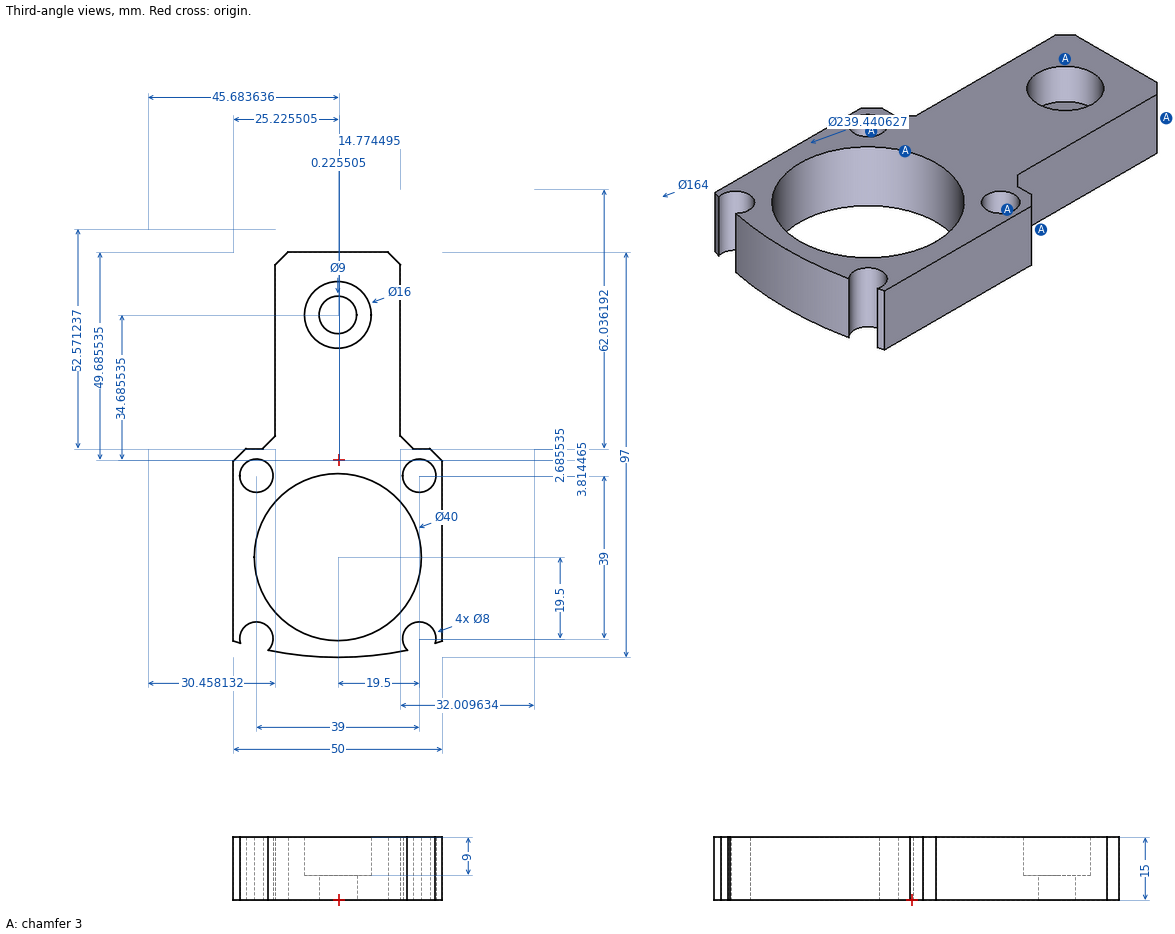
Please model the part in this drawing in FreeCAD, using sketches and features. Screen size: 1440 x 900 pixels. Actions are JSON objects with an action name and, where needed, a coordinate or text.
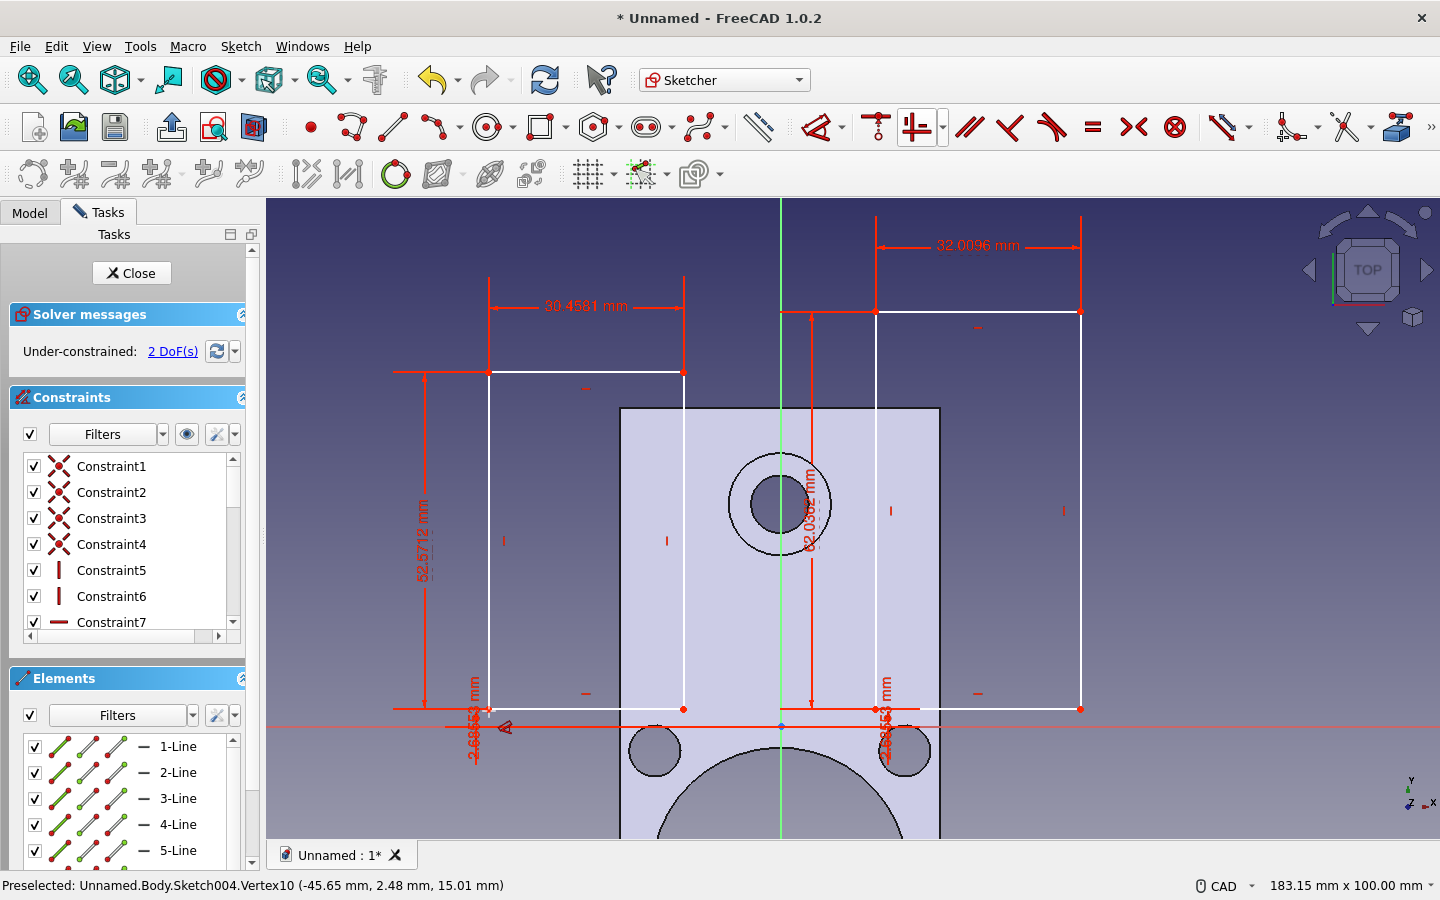
{"action": "left_click", "coordinate": [876, 312]}
{"action": "left_click", "coordinate": [828, 278]}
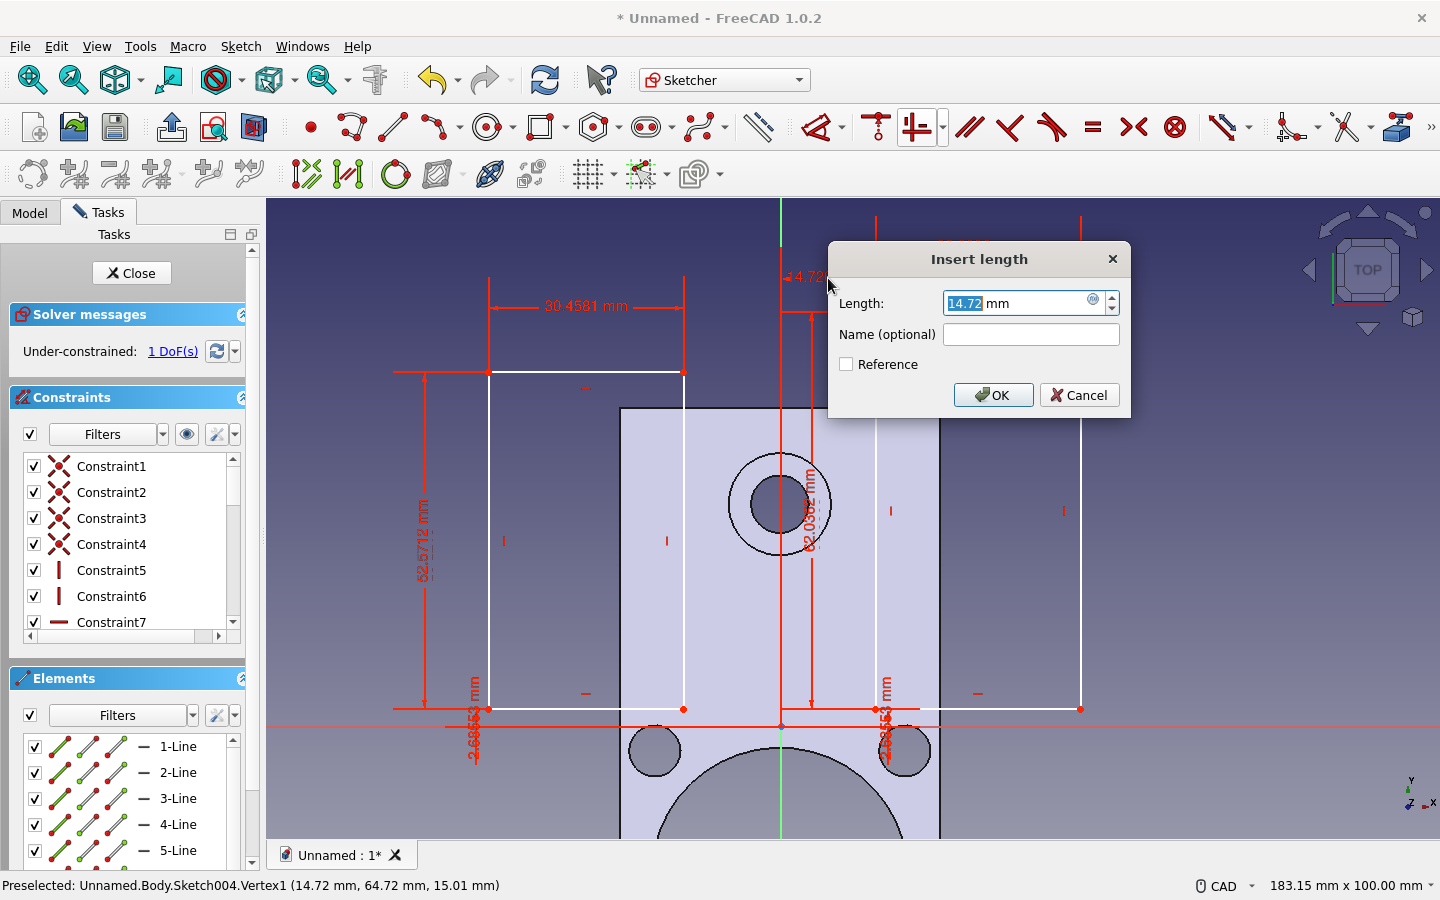
{"action": "type", "text": "14.774495"}
{"action": "key", "text": "Return"}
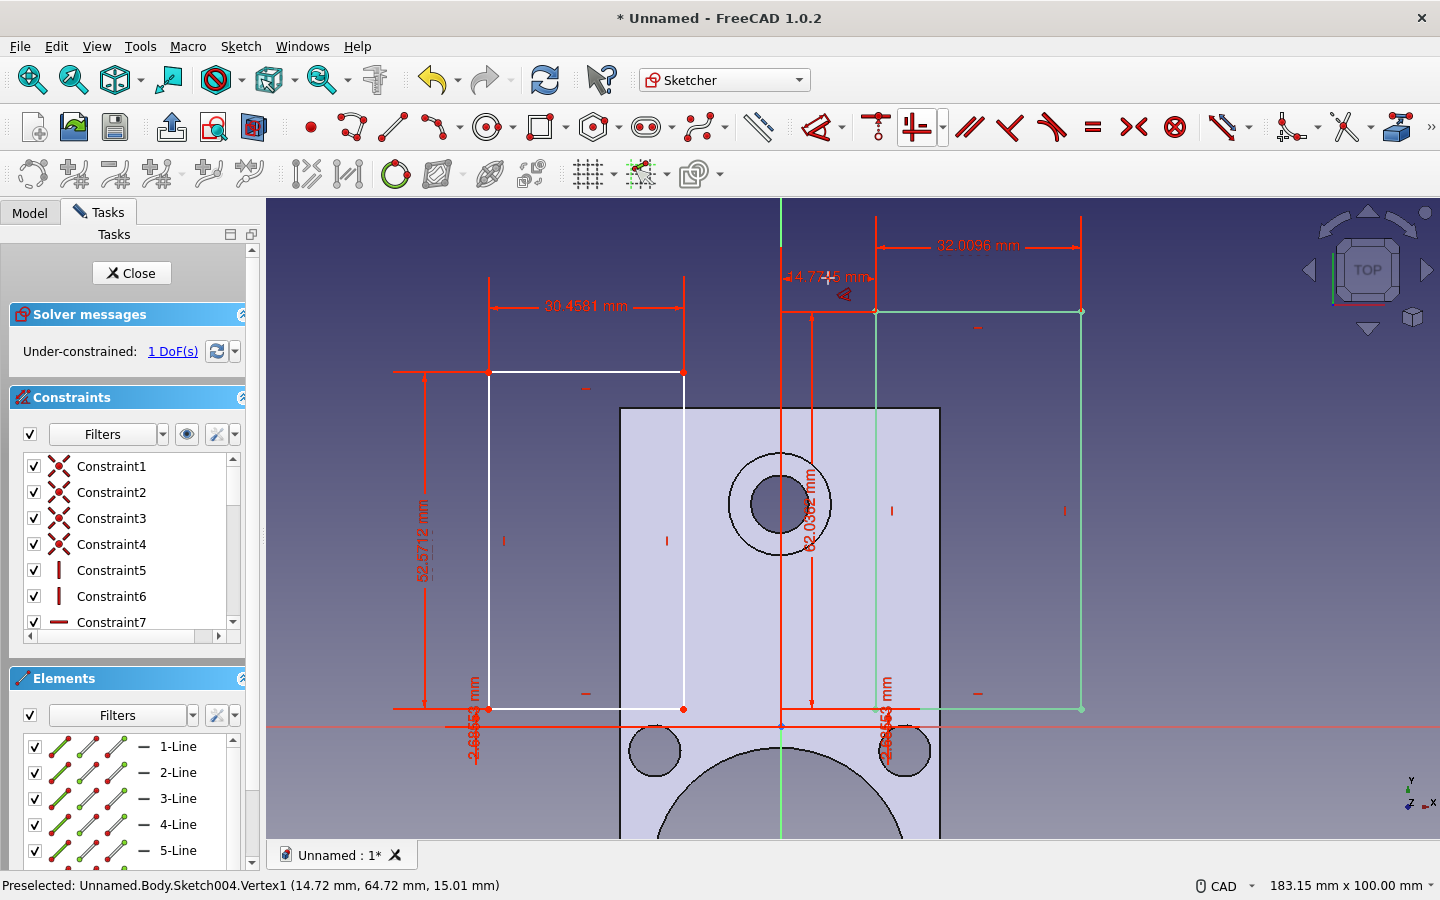
{"action": "left_click", "coordinate": [489, 372]}
{"action": "left_click", "coordinate": [635, 761]}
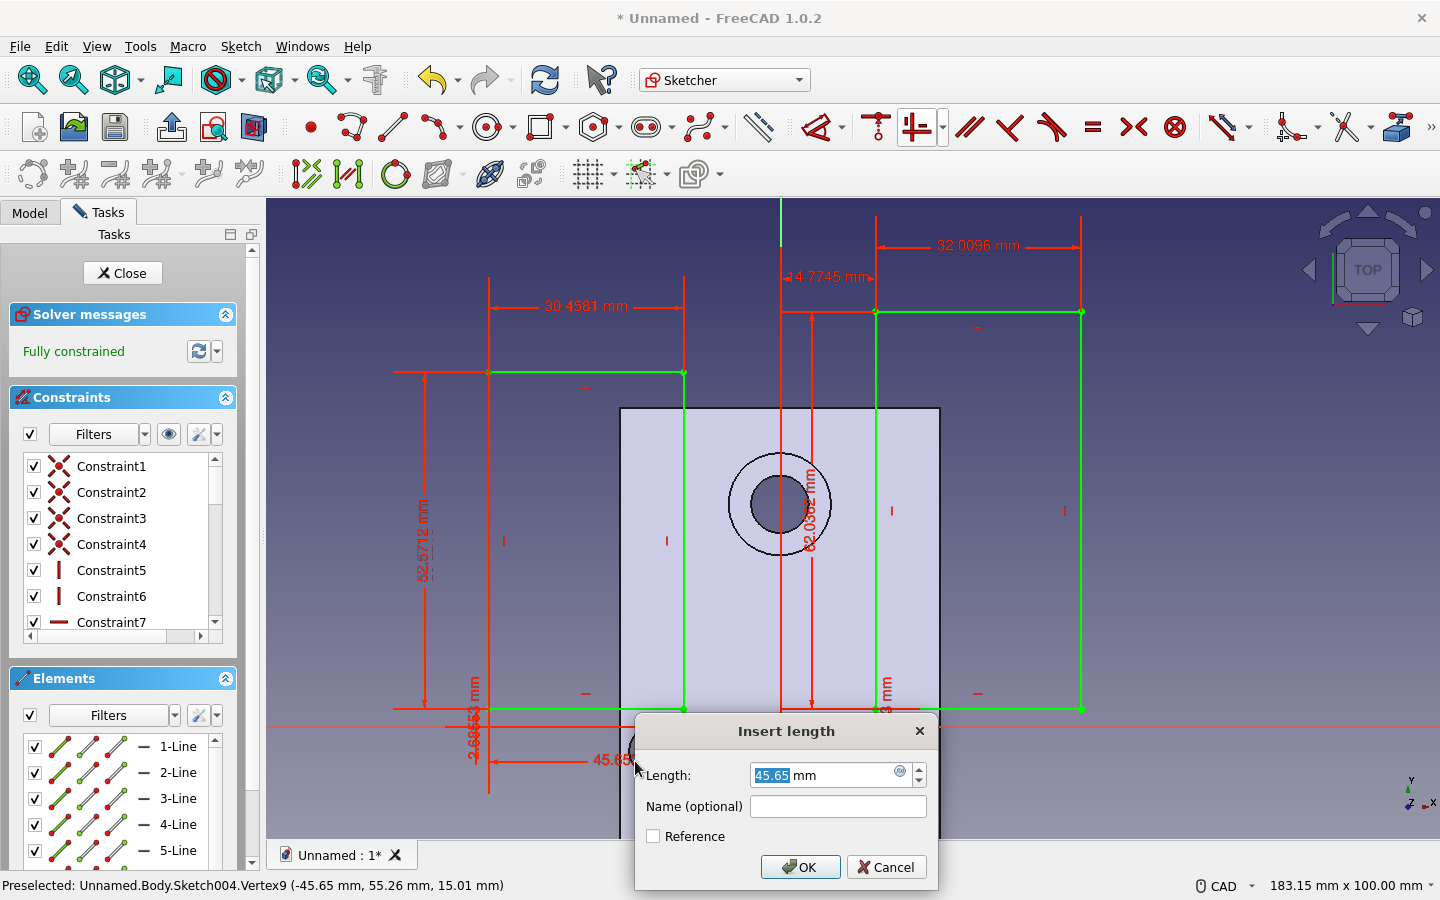
{"action": "type", "text": "45.683636"}
{"action": "key", "text": "Return"}
{"action": "key", "text": "Escape"}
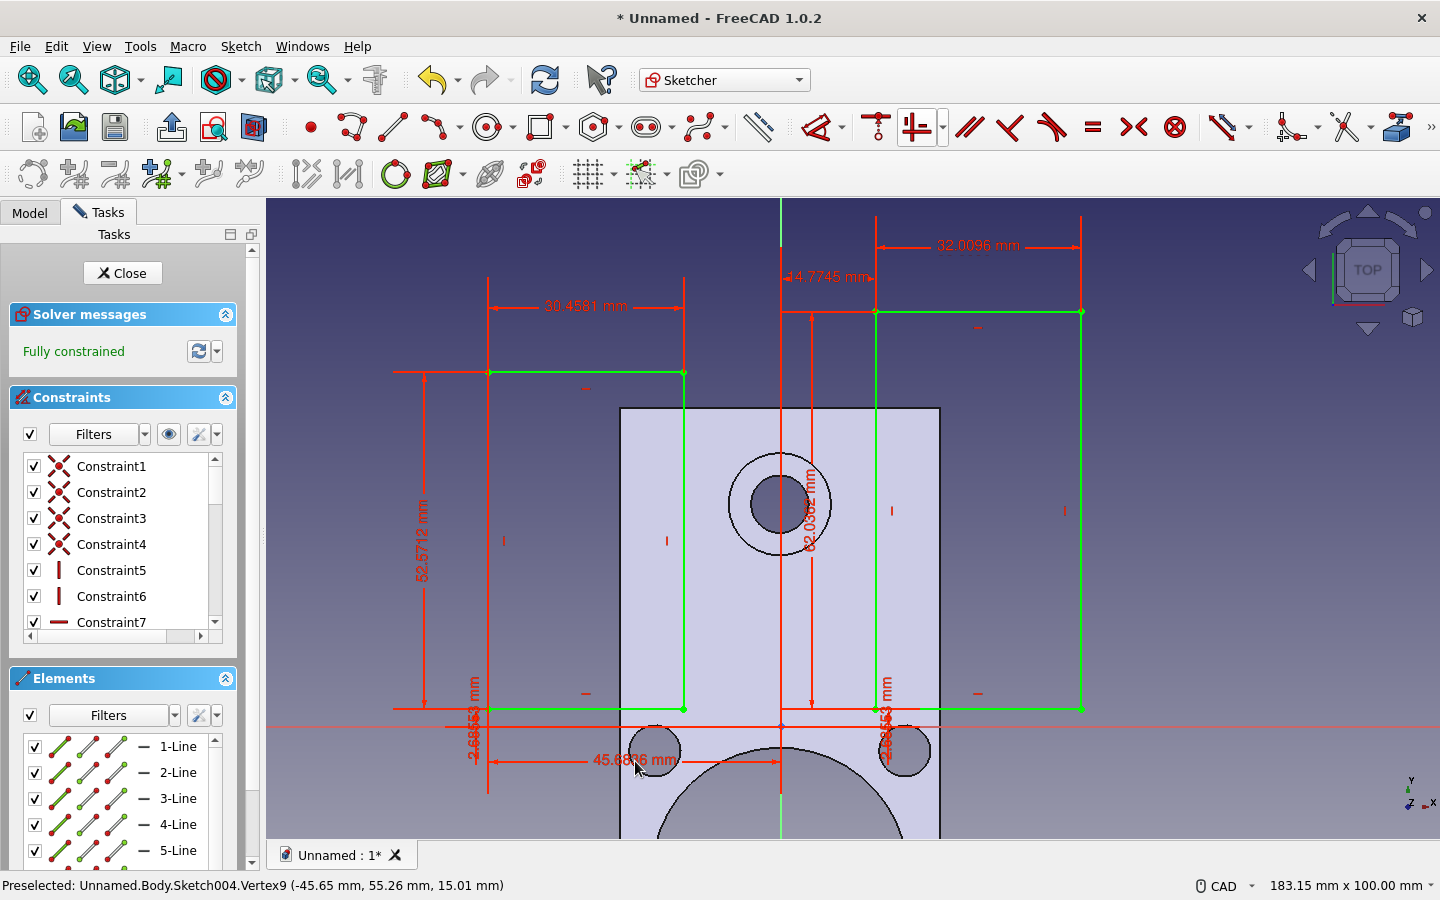
{"action": "left_click", "coordinate": [123, 273]}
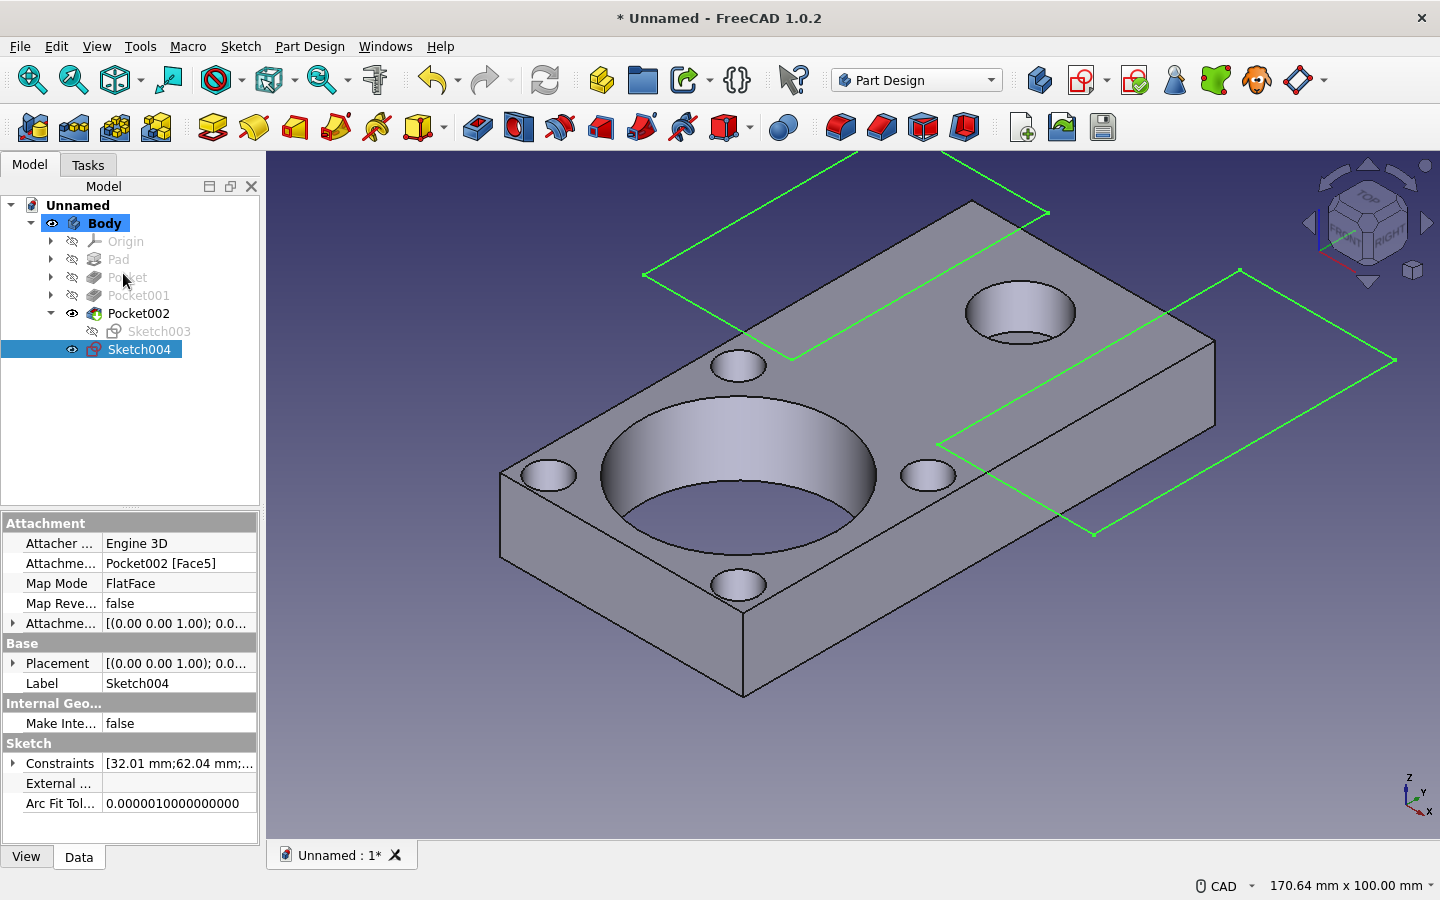
{"action": "left_click", "coordinate": [478, 128]}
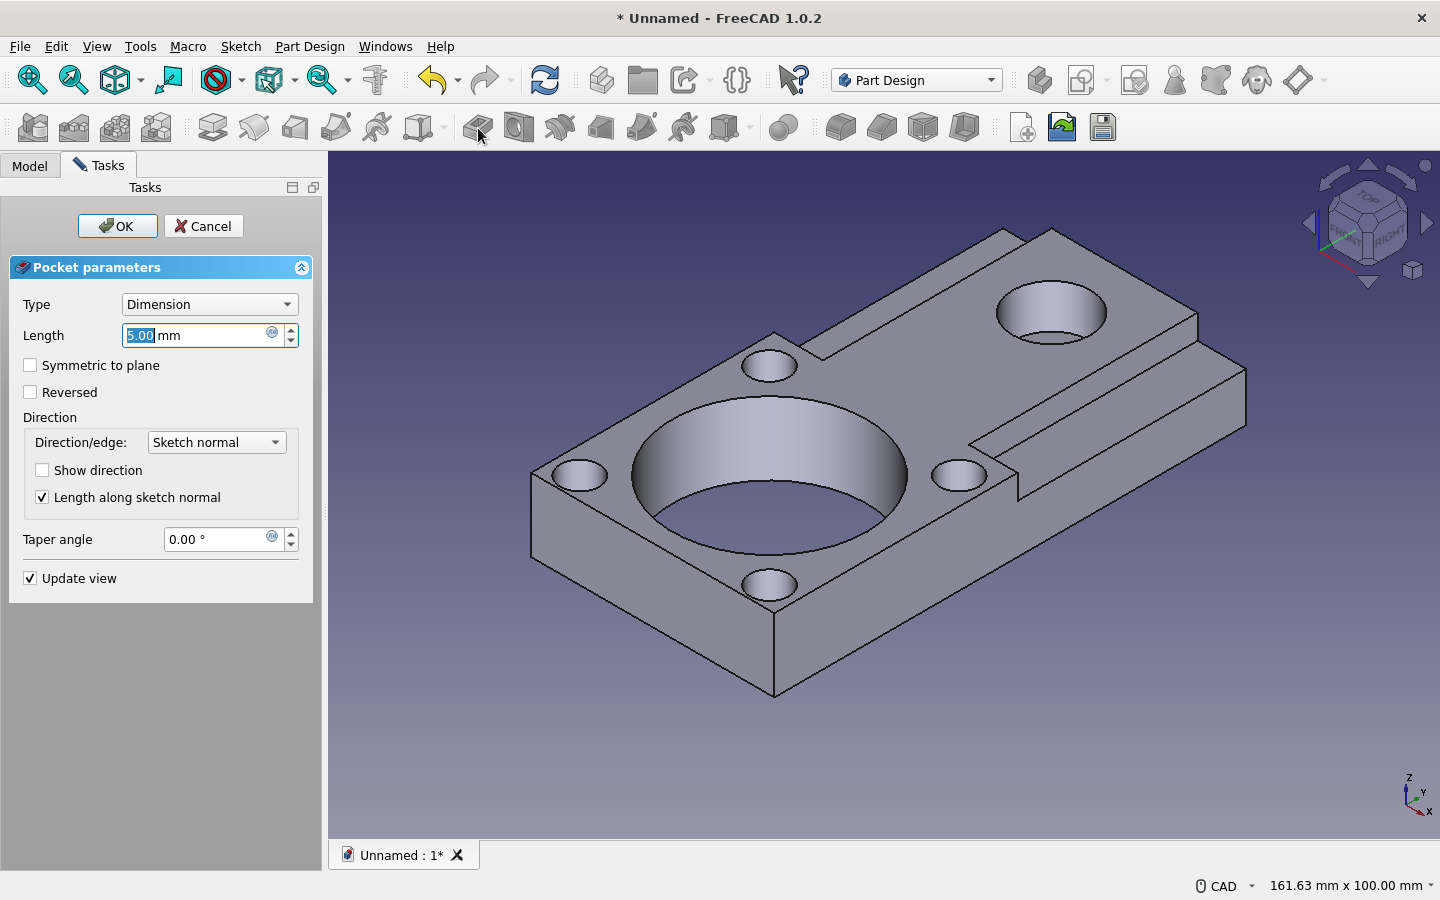
{"action": "left_click", "coordinate": [210, 304]}